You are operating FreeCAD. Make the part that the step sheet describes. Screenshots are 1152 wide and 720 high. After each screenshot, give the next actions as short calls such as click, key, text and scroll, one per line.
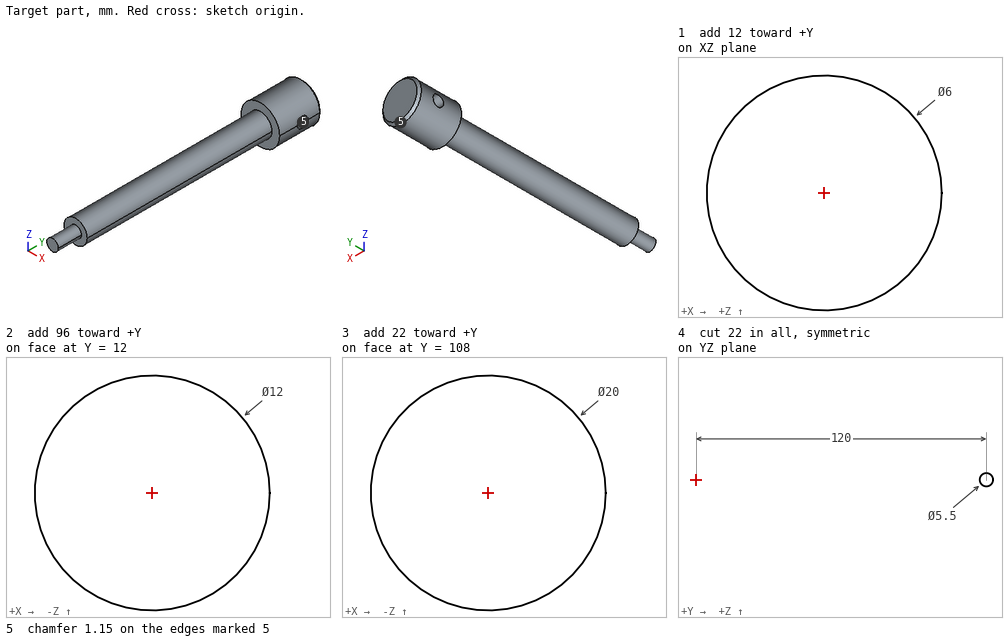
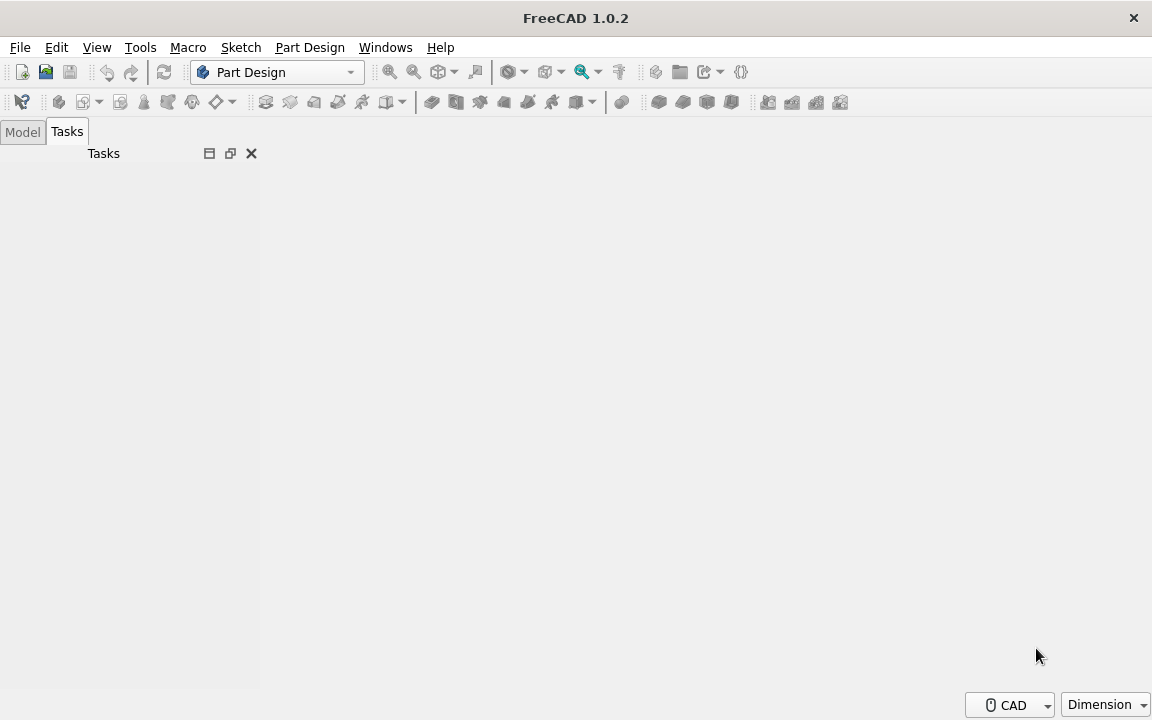
click(22, 72)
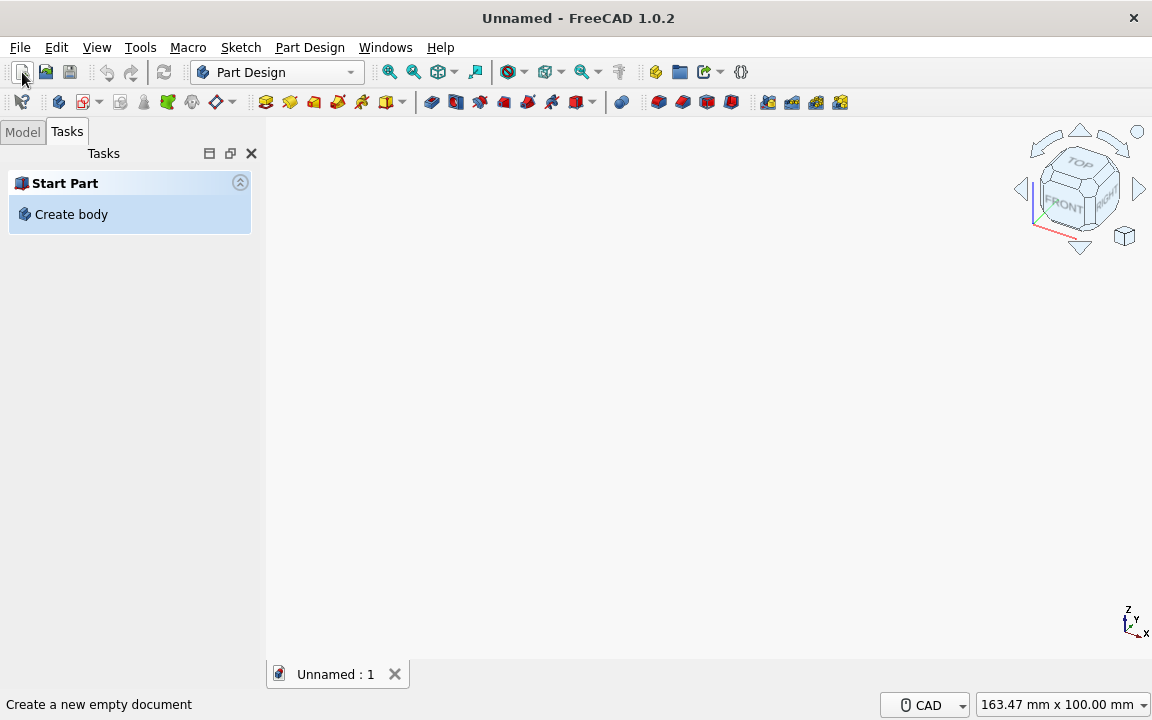
click(84, 102)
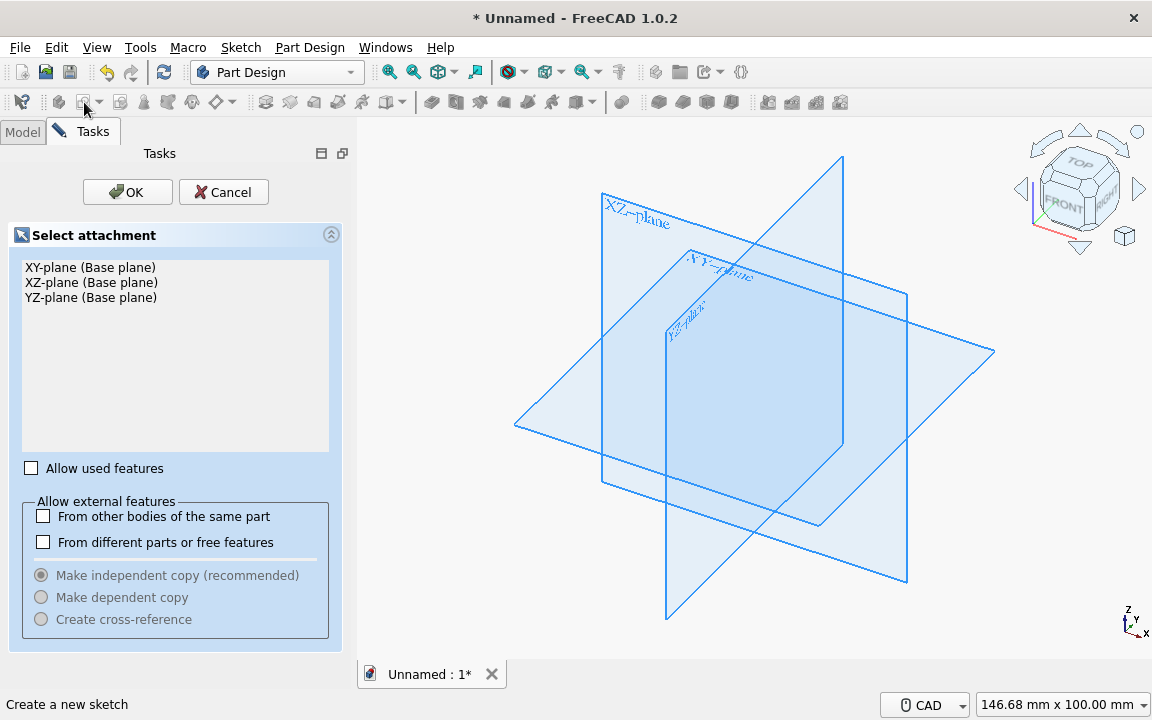
click(82, 282)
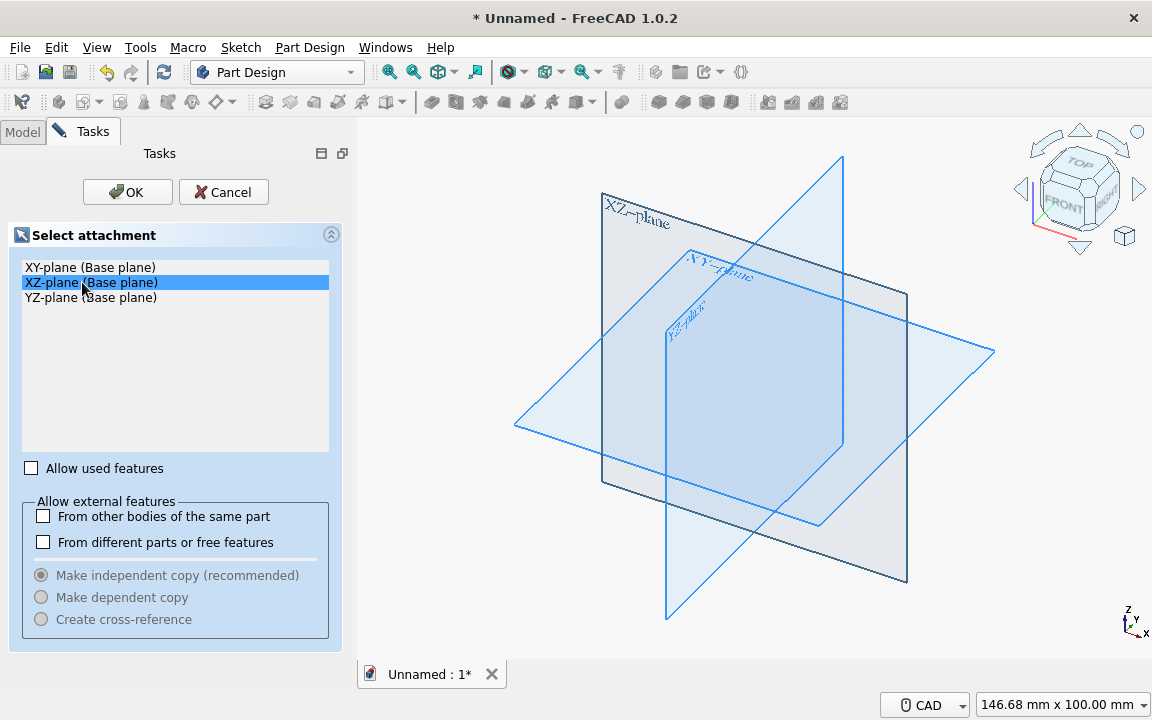
click(128, 192)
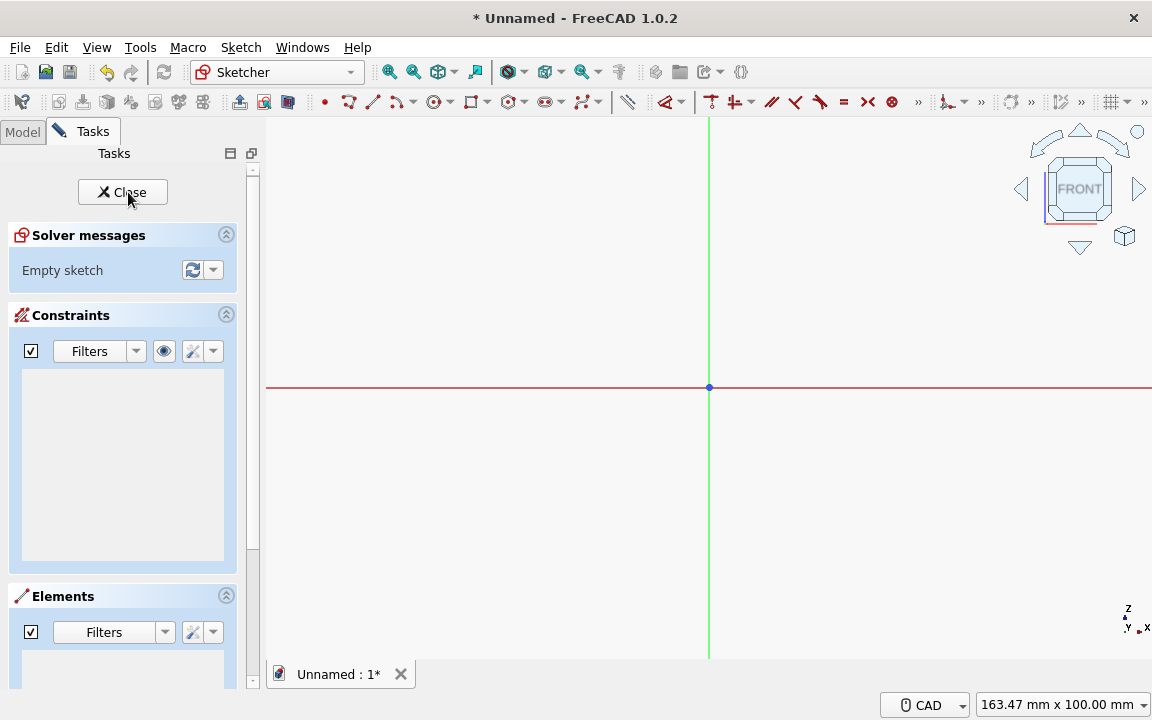
scroll(716, 388, up, 12)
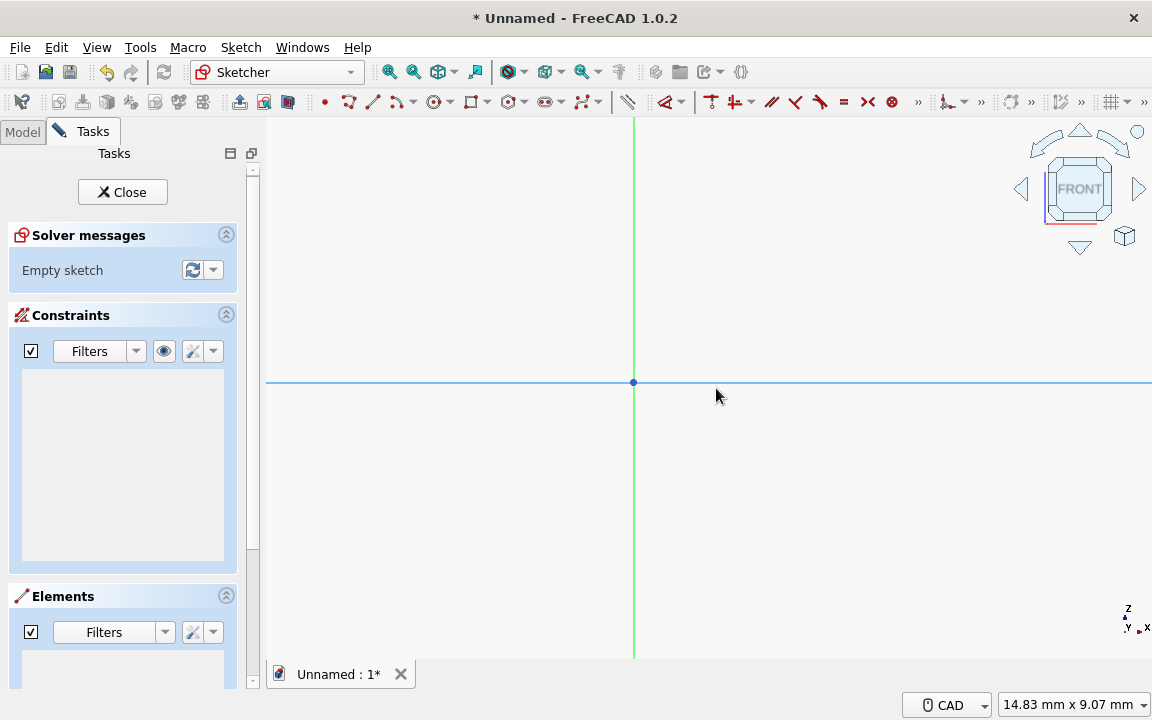
click(434, 102)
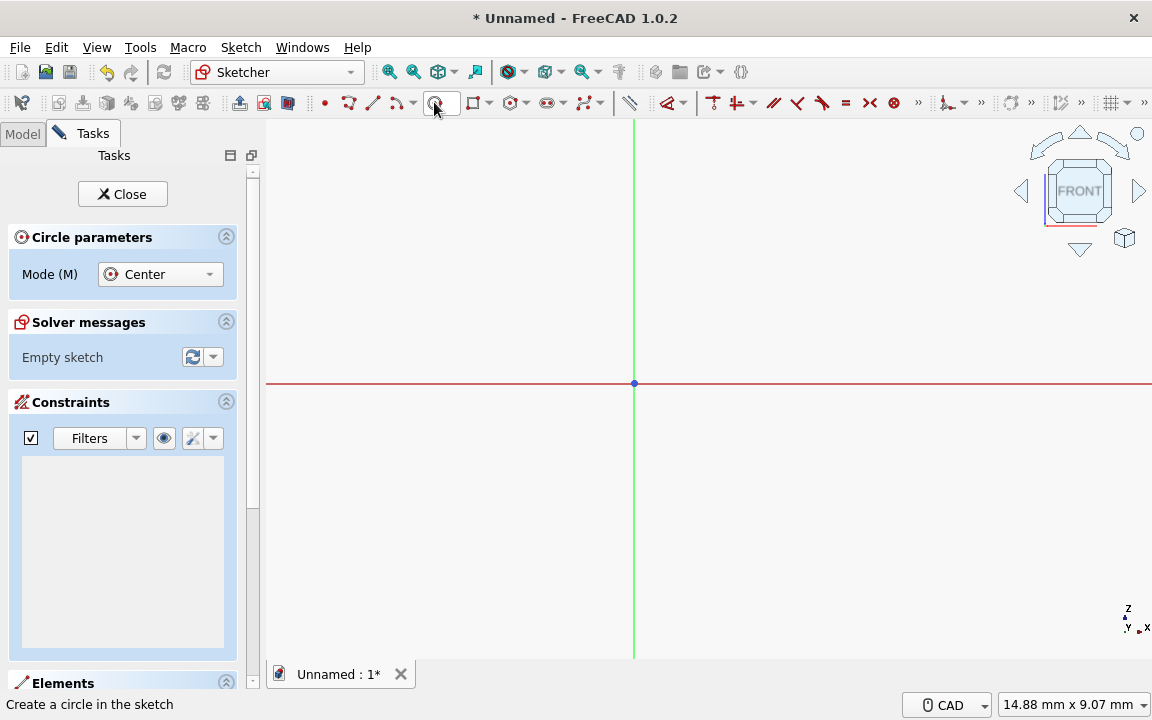
click(634, 384)
move(760, 258)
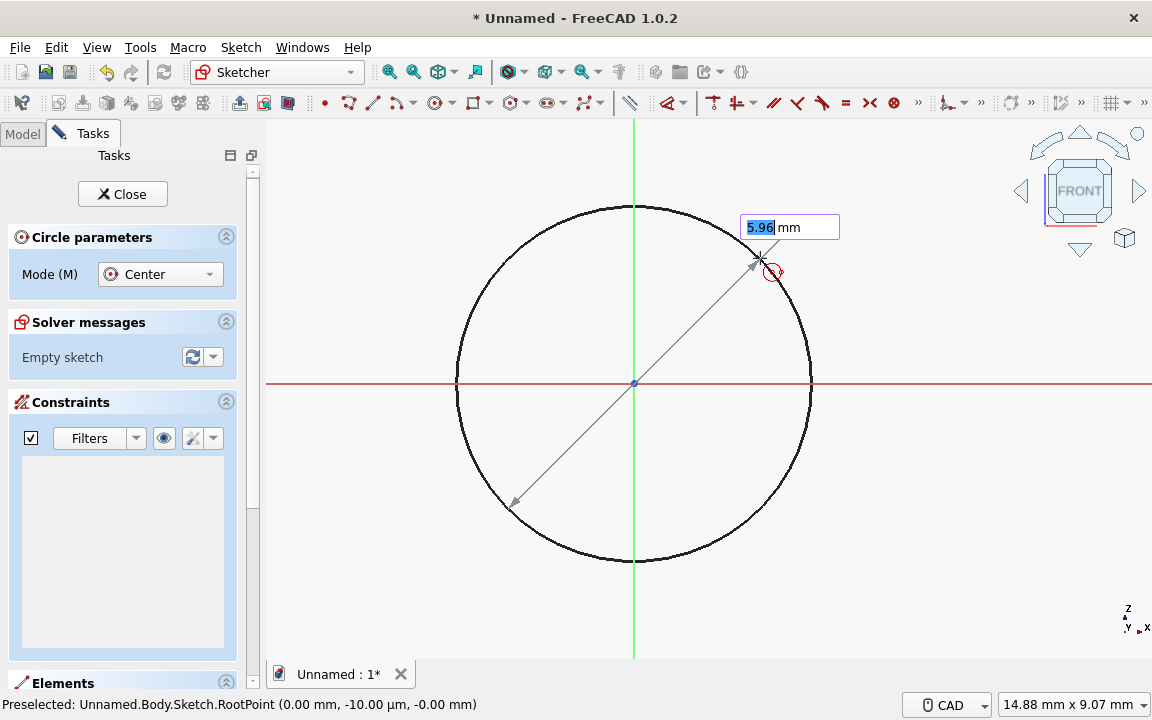
text(6)
key(Return)
key(Escape)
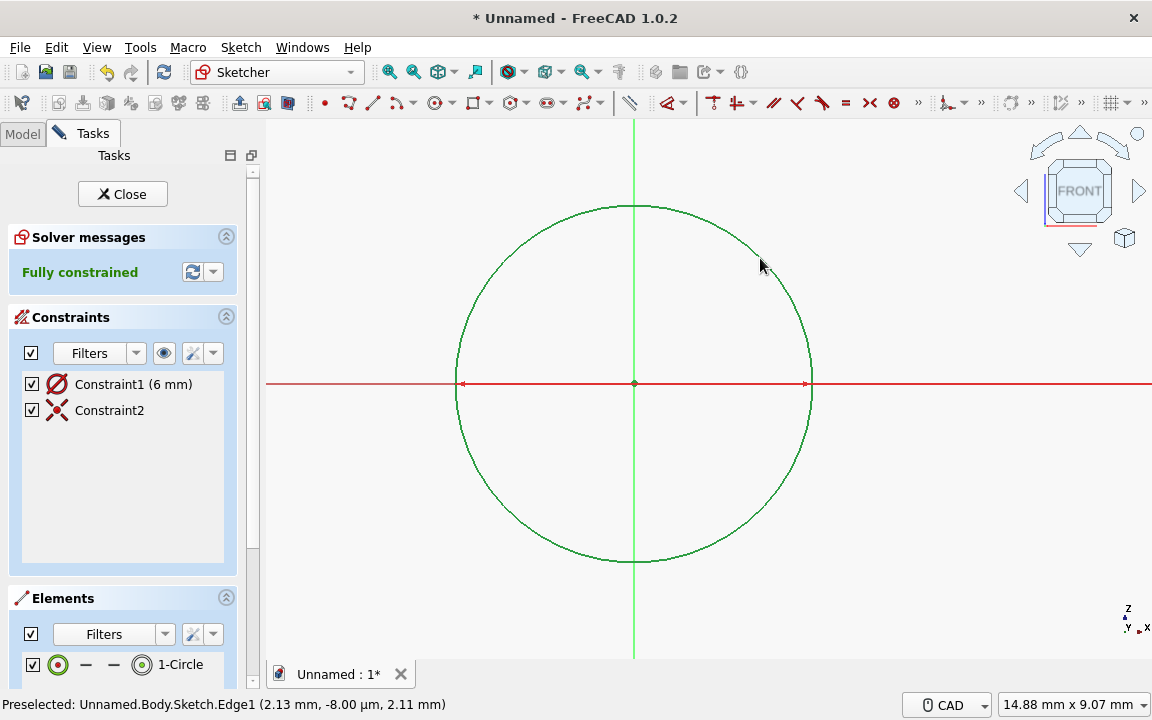
click(123, 194)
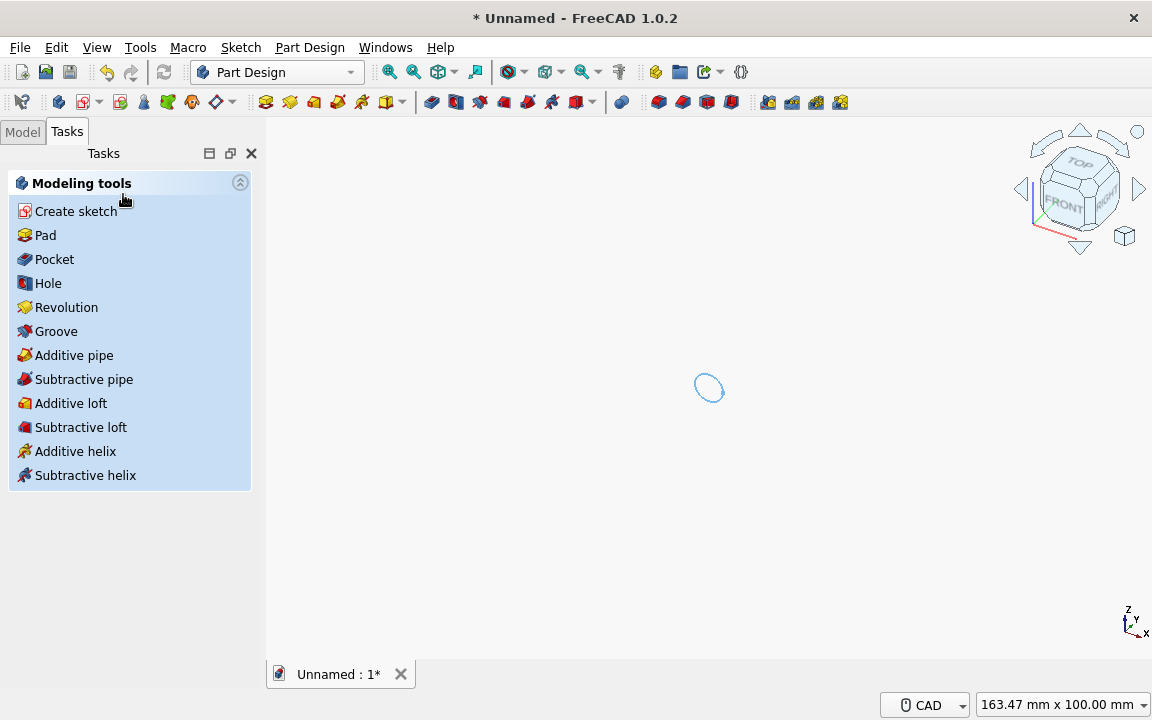
click(266, 102)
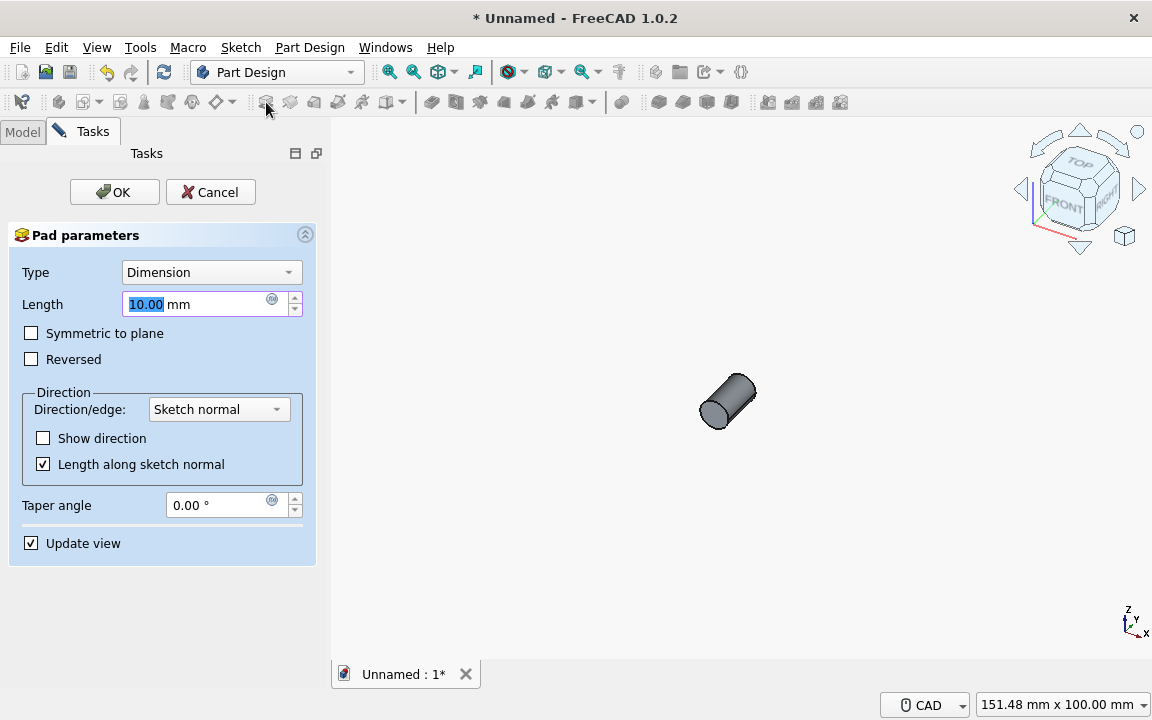
text(12)
key(Tab)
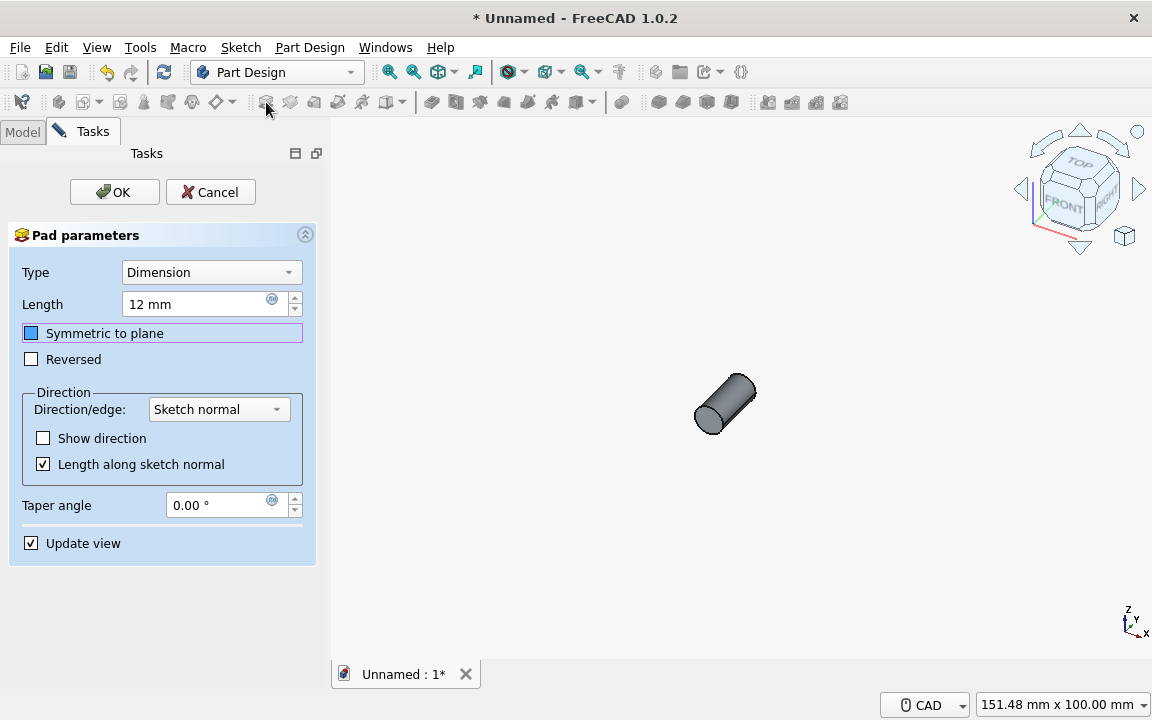
click(30, 359)